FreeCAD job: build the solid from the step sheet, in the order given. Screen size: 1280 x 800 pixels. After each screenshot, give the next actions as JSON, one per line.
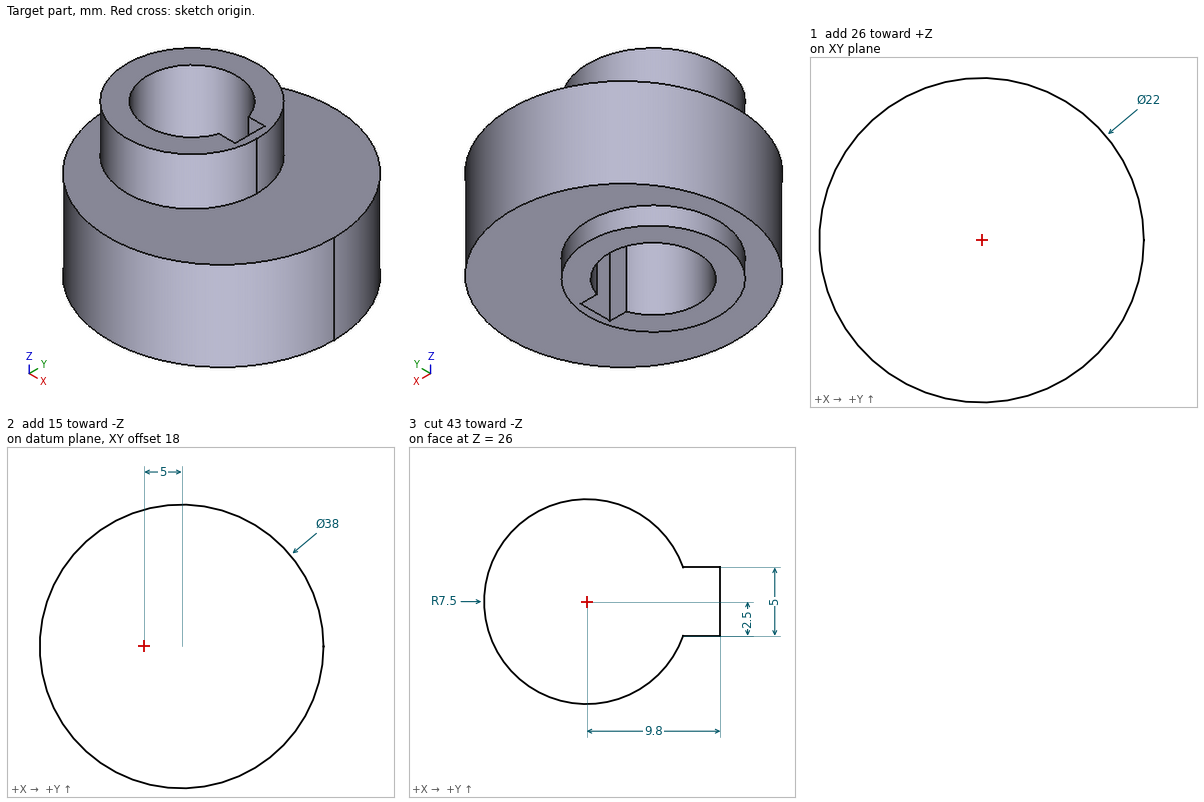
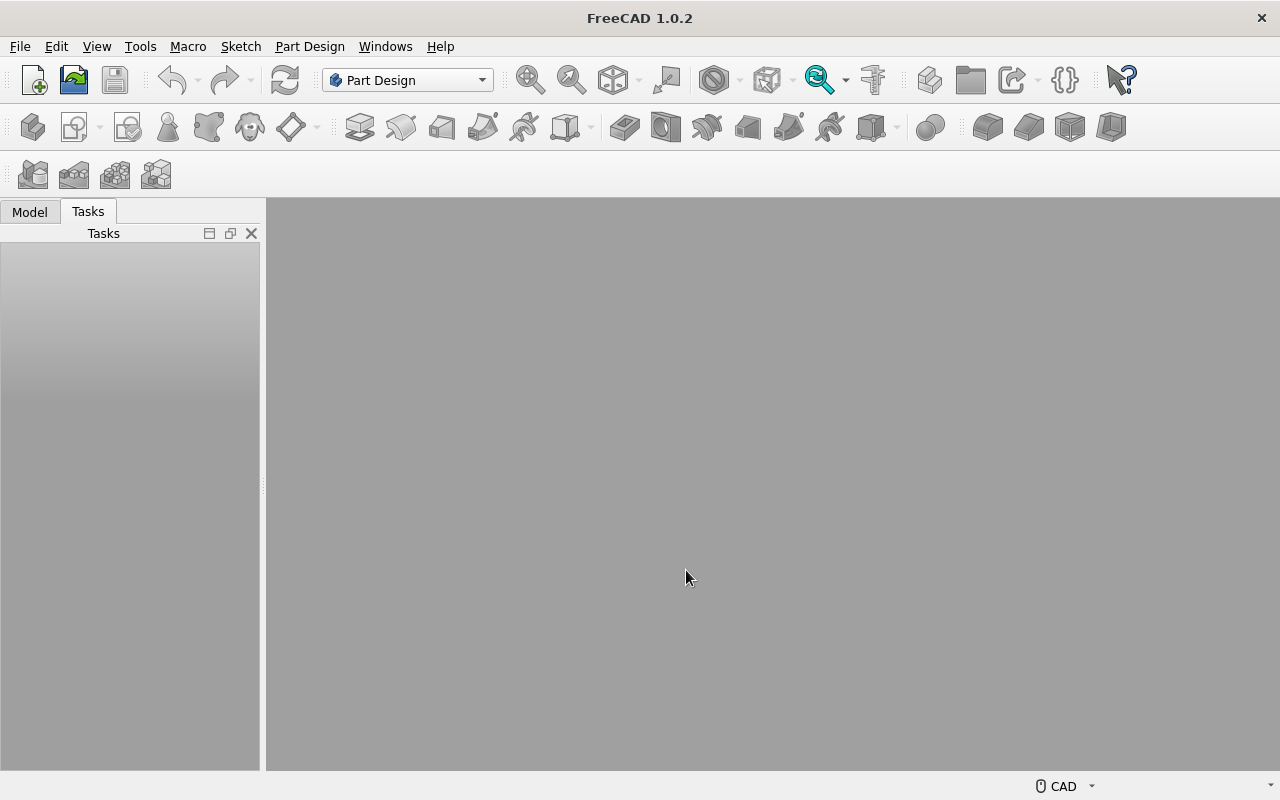
{"action": "left_click", "coordinate": [33, 80]}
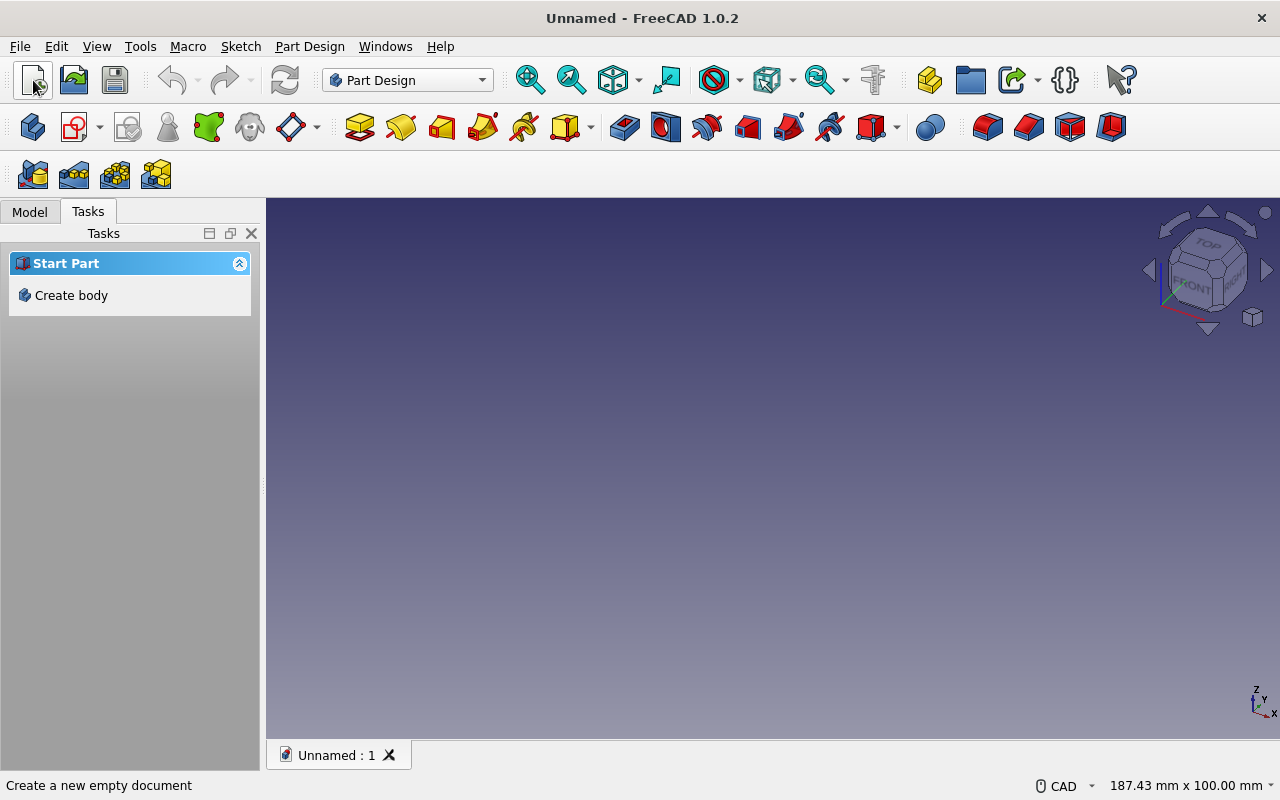
{"action": "left_click", "coordinate": [74, 128]}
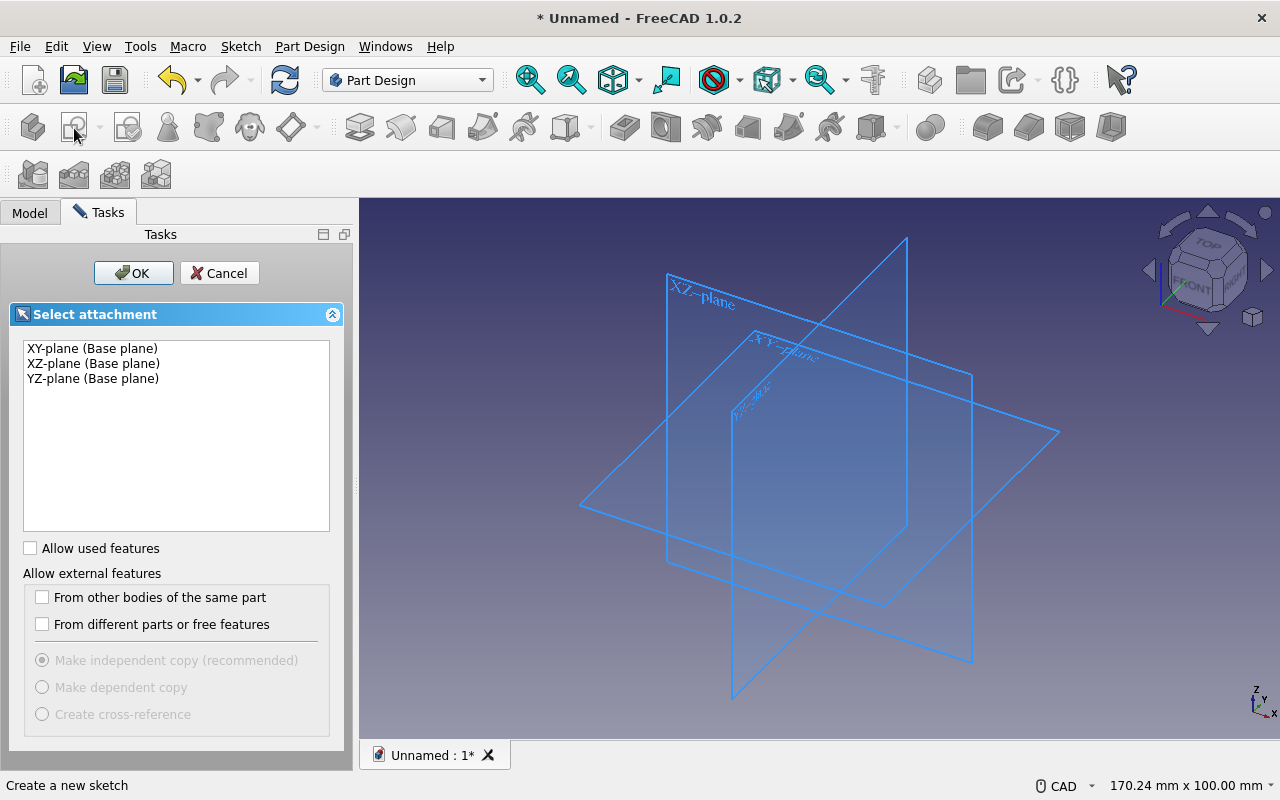
{"action": "left_click", "coordinate": [84, 348]}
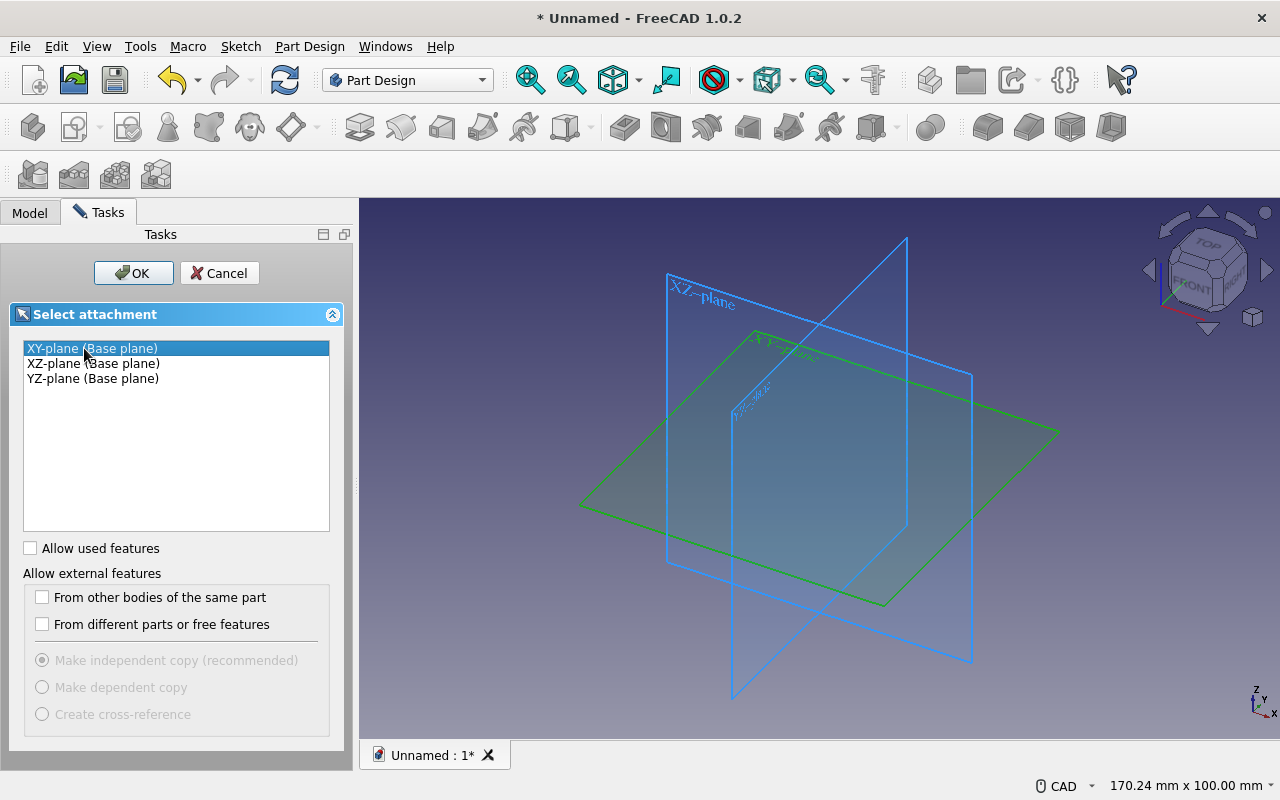
{"action": "left_click", "coordinate": [134, 273]}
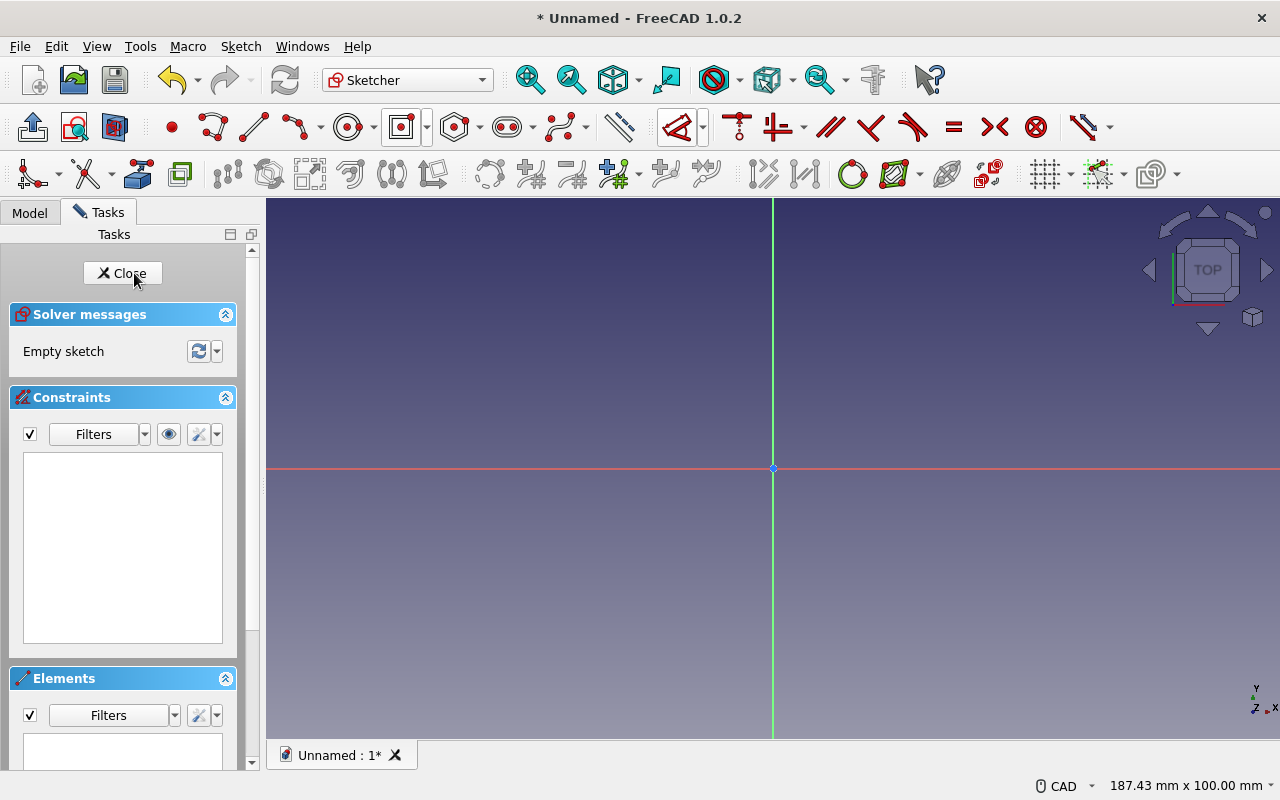
{"action": "scroll", "coordinate": [813, 468], "scroll_direction": "up", "scroll_amount": 5}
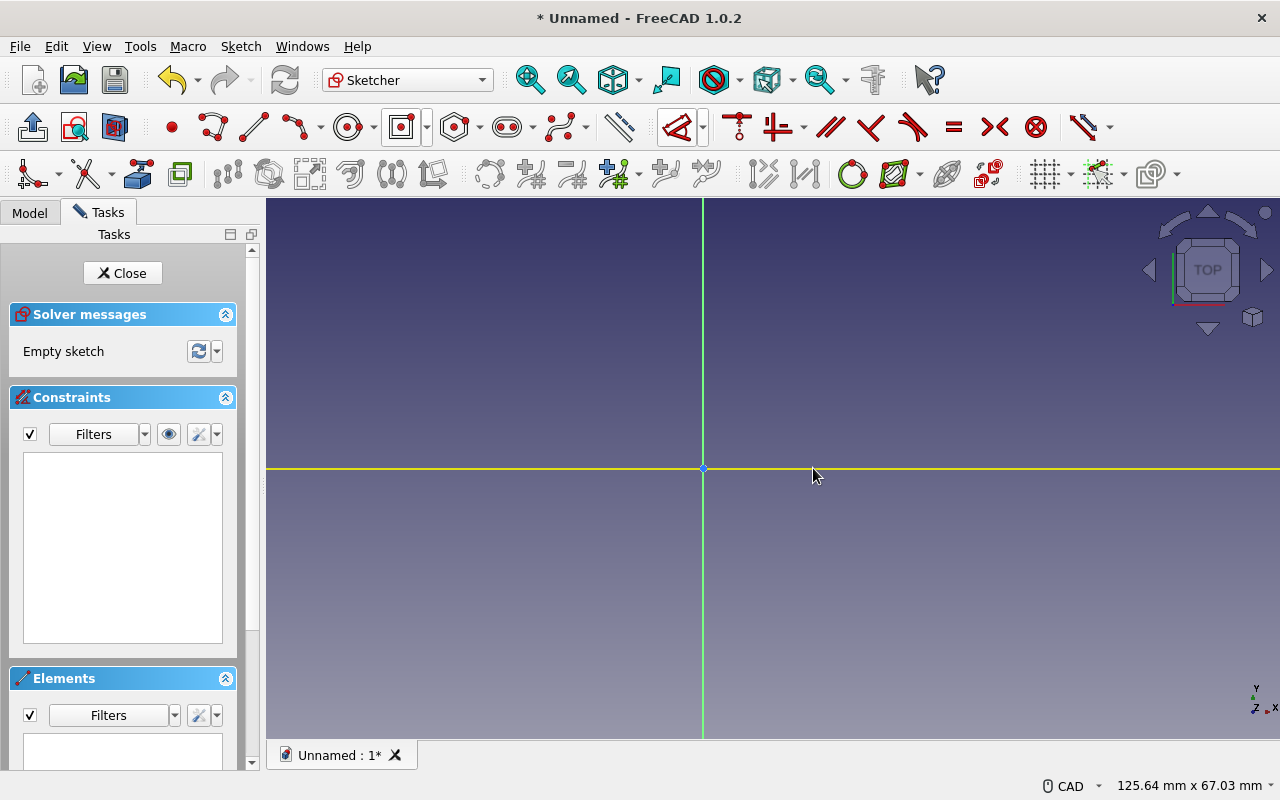
{"action": "left_click", "coordinate": [348, 128]}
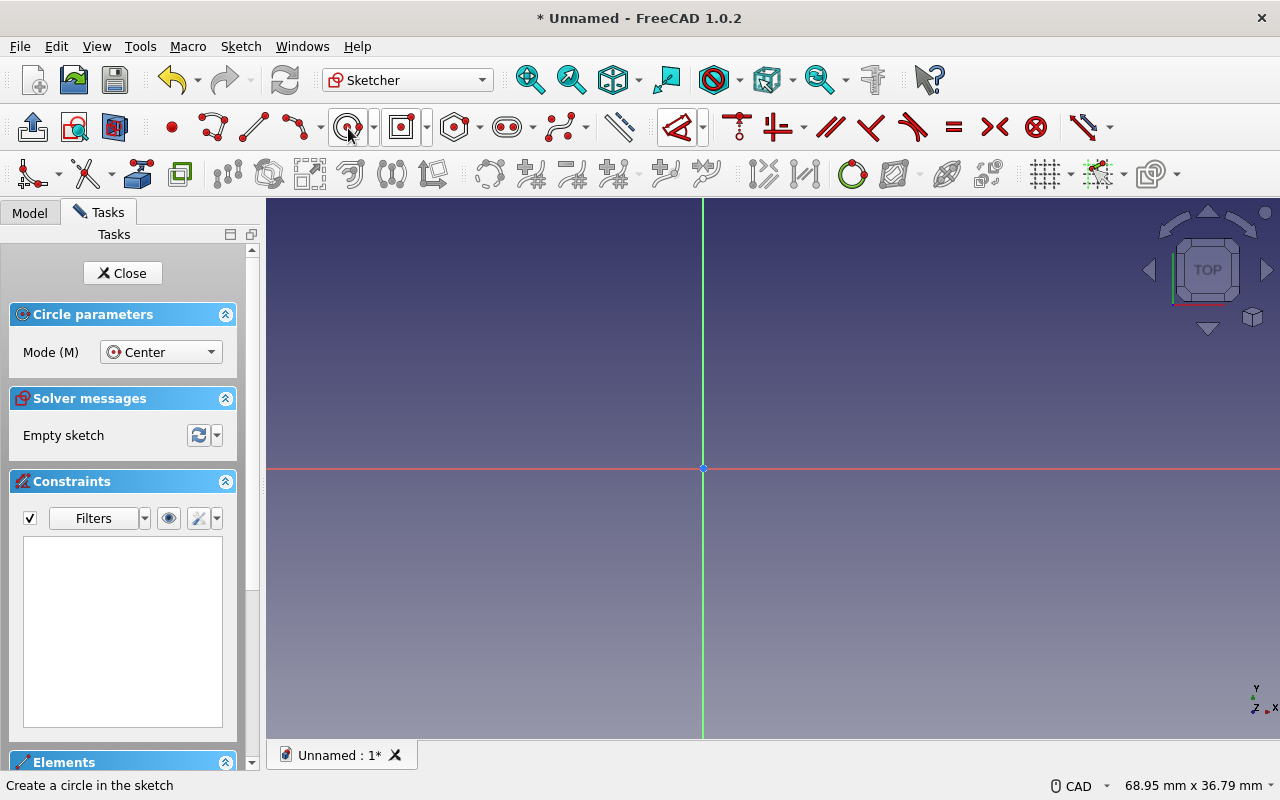
{"action": "left_click", "coordinate": [703, 468]}
{"action": "left_click", "coordinate": [818, 354]}
{"action": "key", "text": "Escape"}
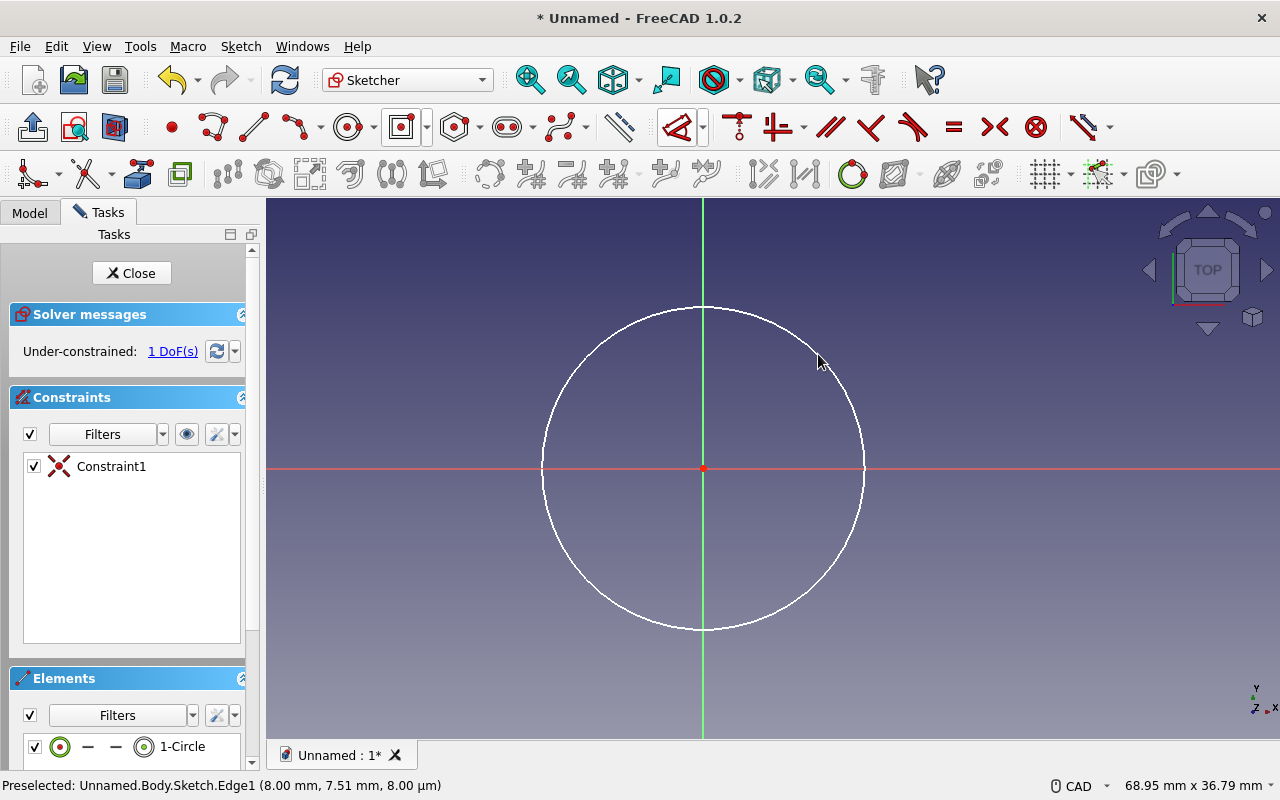
{"action": "key", "text": "d"}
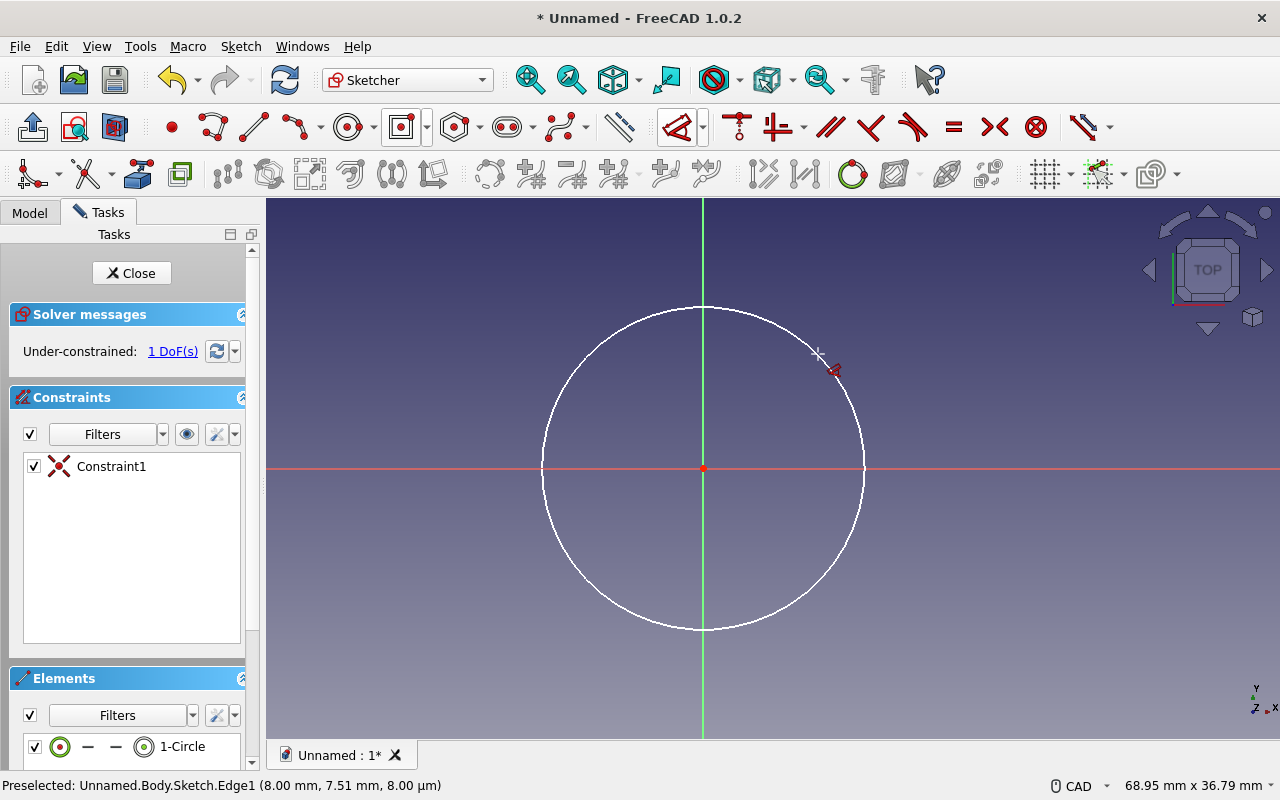
{"action": "left_click", "coordinate": [817, 354]}
{"action": "left_click", "coordinate": [840, 331]}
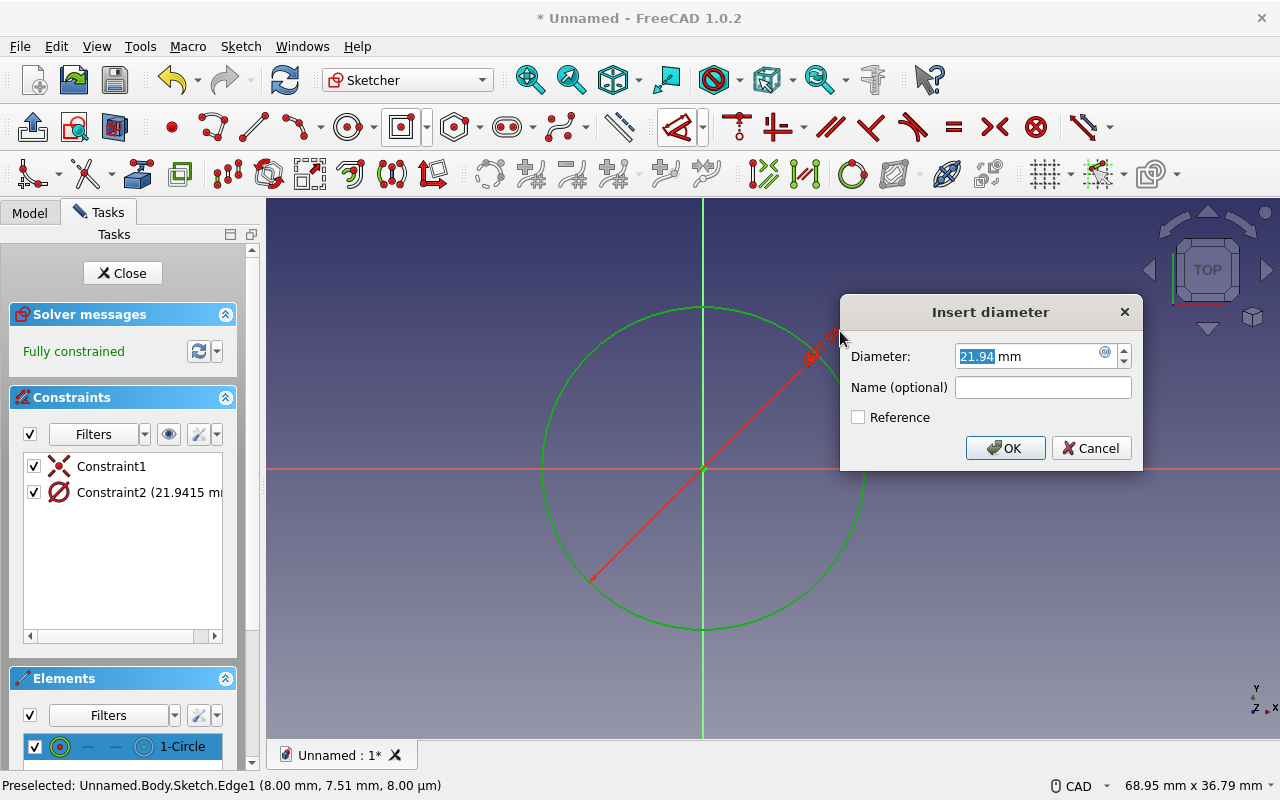
{"action": "type", "text": "22"}
{"action": "key", "text": "Return"}
{"action": "key", "text": "Escape"}